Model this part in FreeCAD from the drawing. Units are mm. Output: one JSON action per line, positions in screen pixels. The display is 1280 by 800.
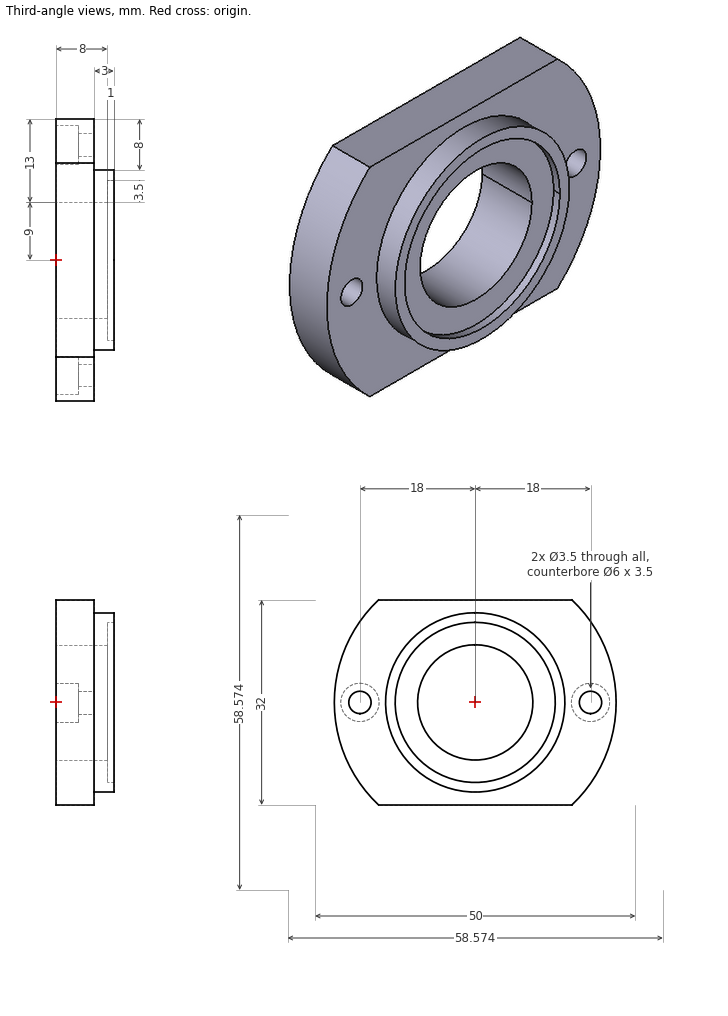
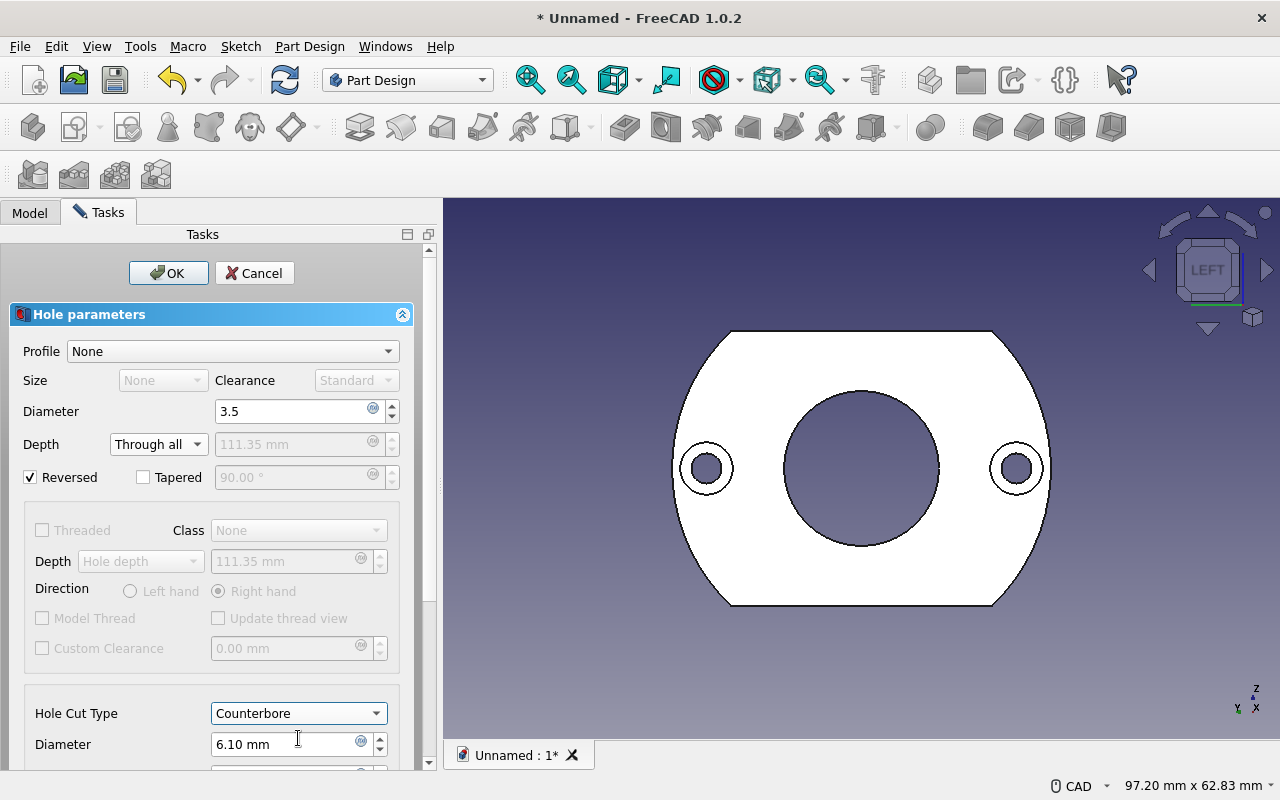
{"action": "triple_click", "coordinate": [292, 744]}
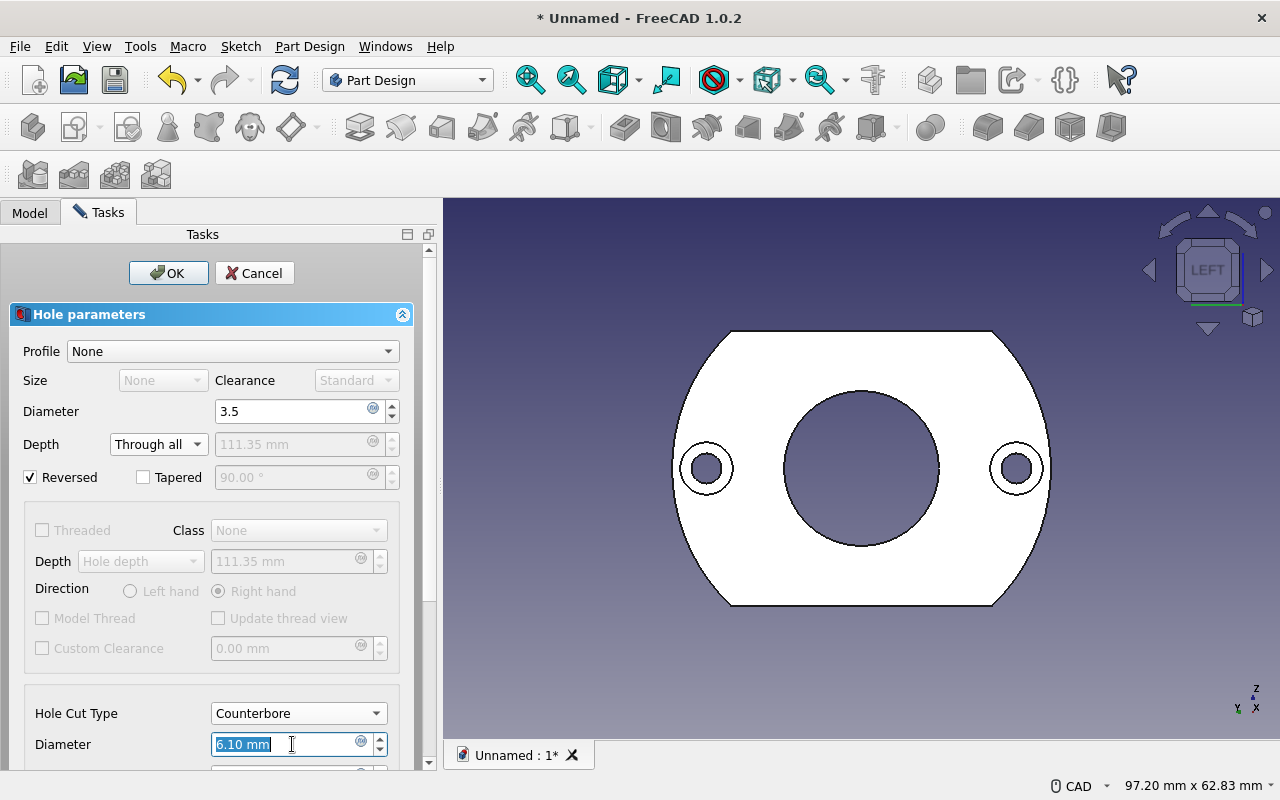
{"action": "type", "text": "6"}
{"action": "key", "text": "Tab"}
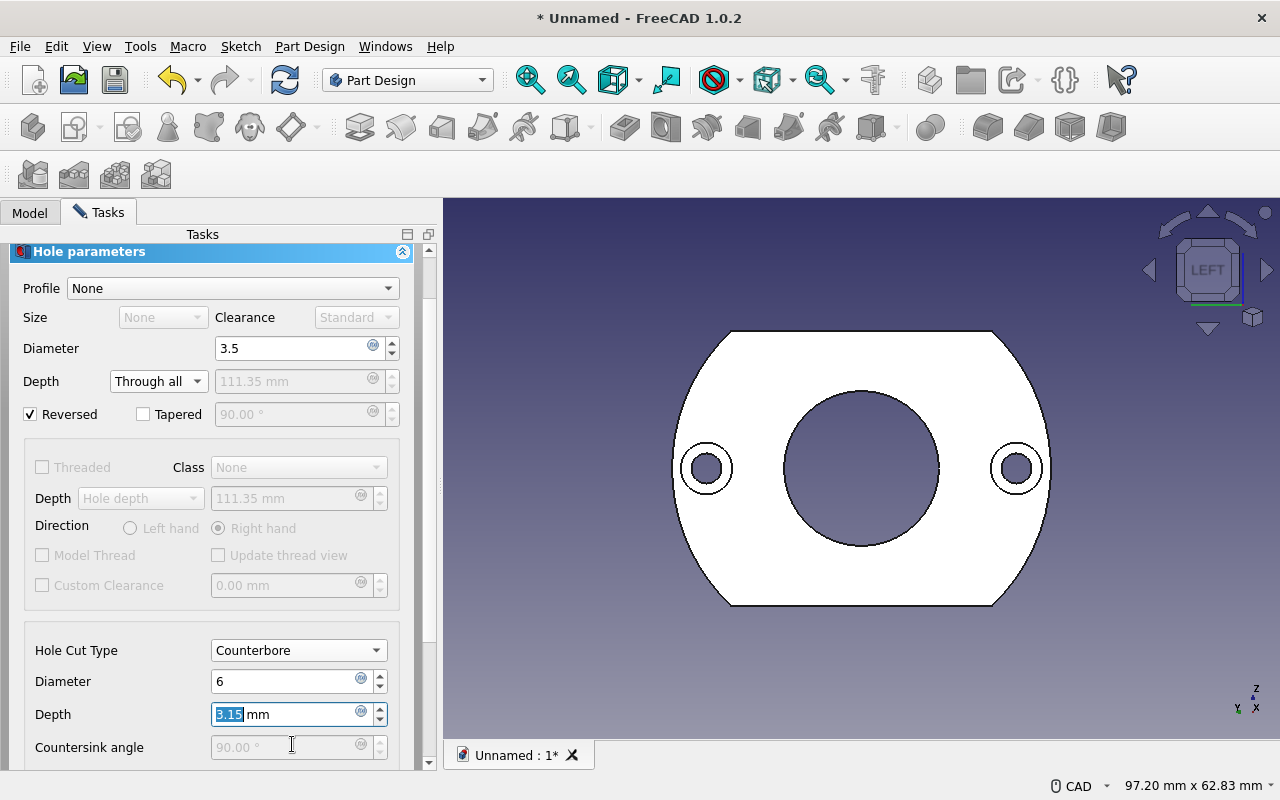
{"action": "type", "text": "3.5"}
{"action": "key", "text": "Tab"}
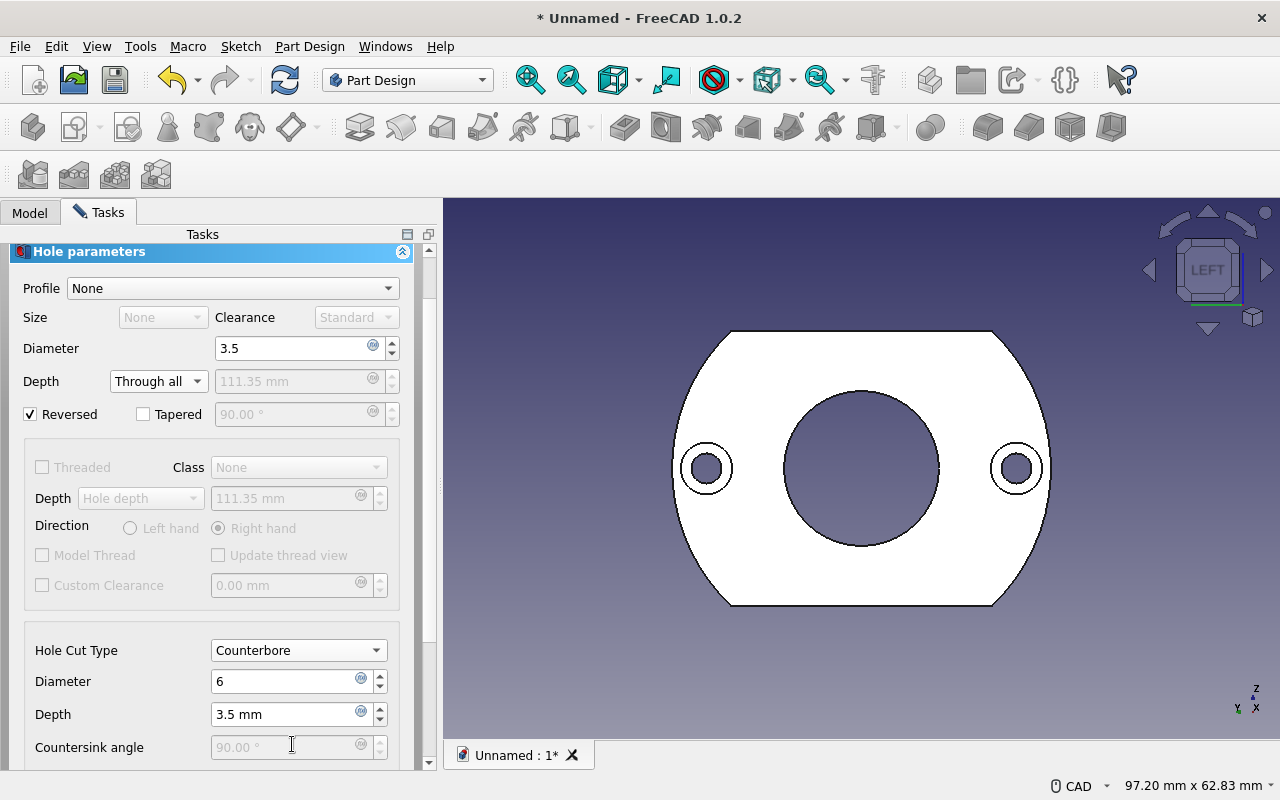
{"action": "scroll", "coordinate": [429, 507], "scroll_direction": "up", "scroll_amount": 2}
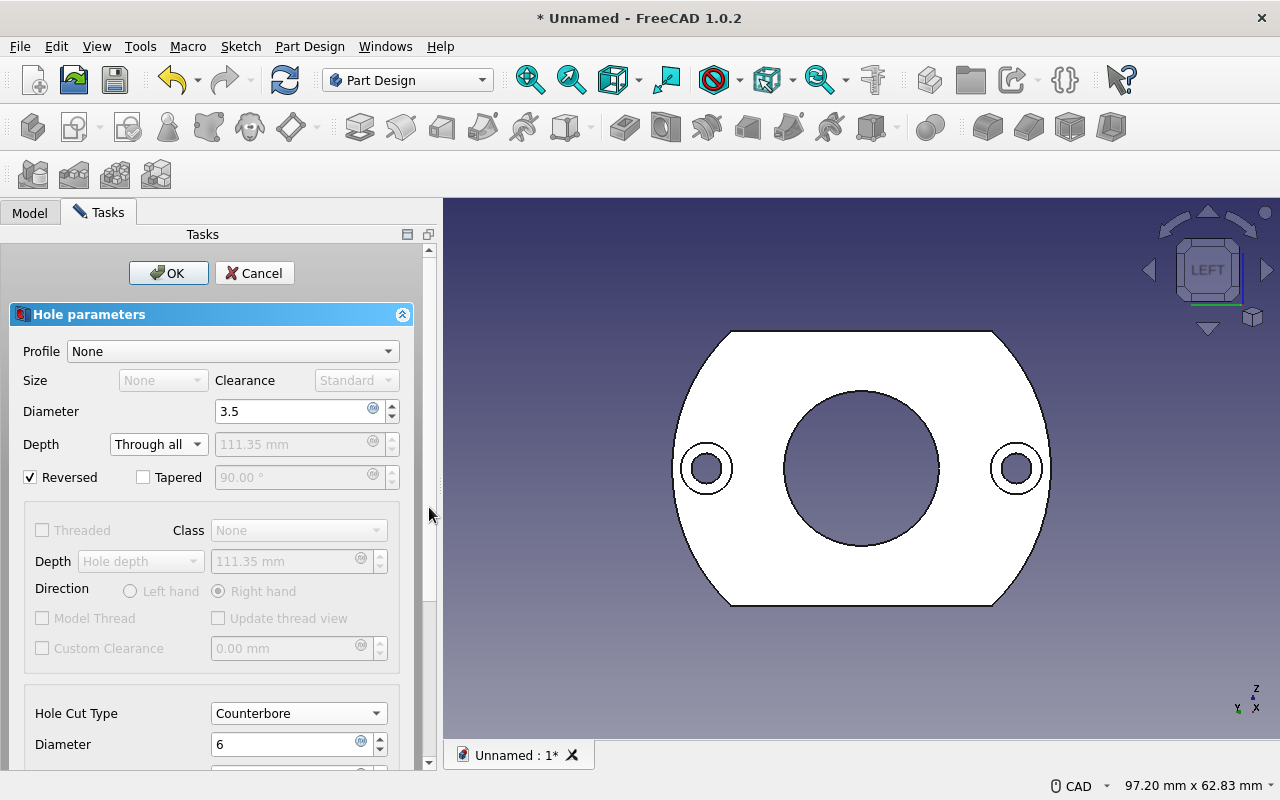
{"action": "left_click", "coordinate": [169, 273]}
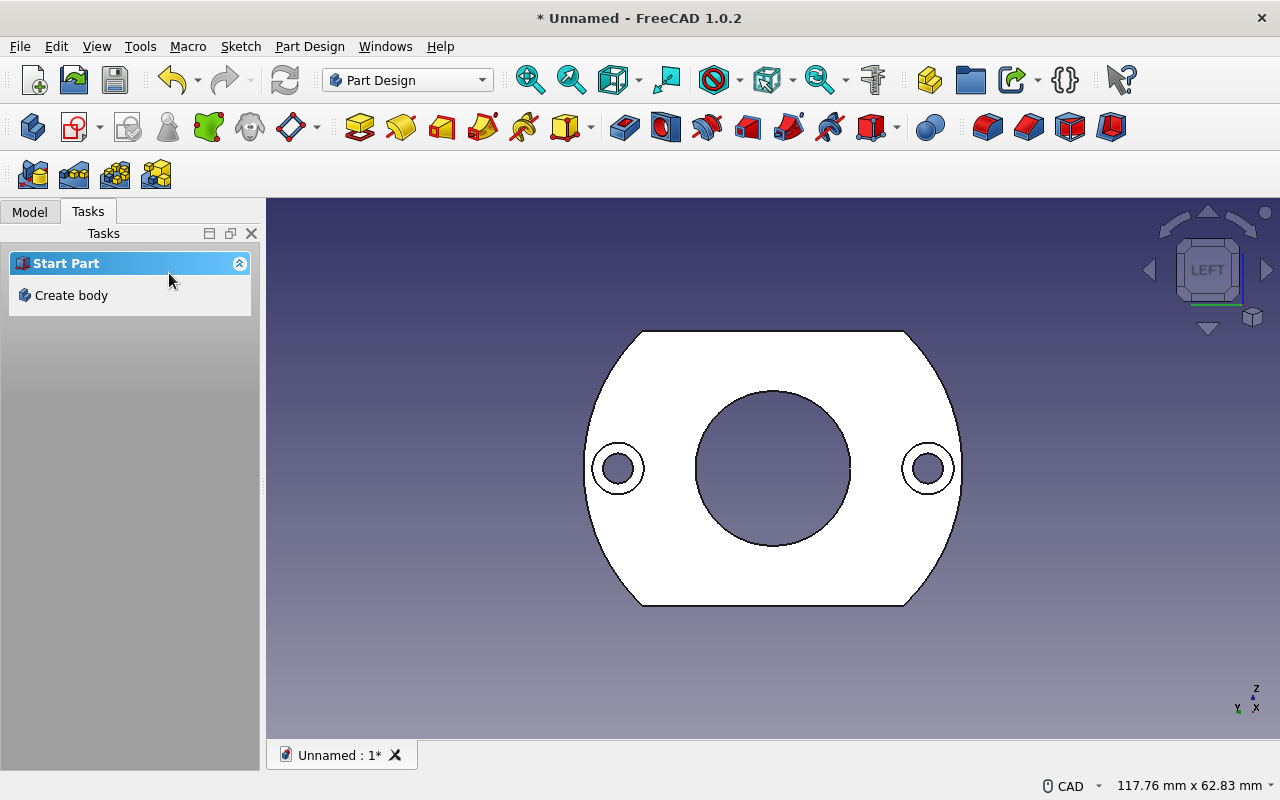
{"action": "key", "text": "0"}